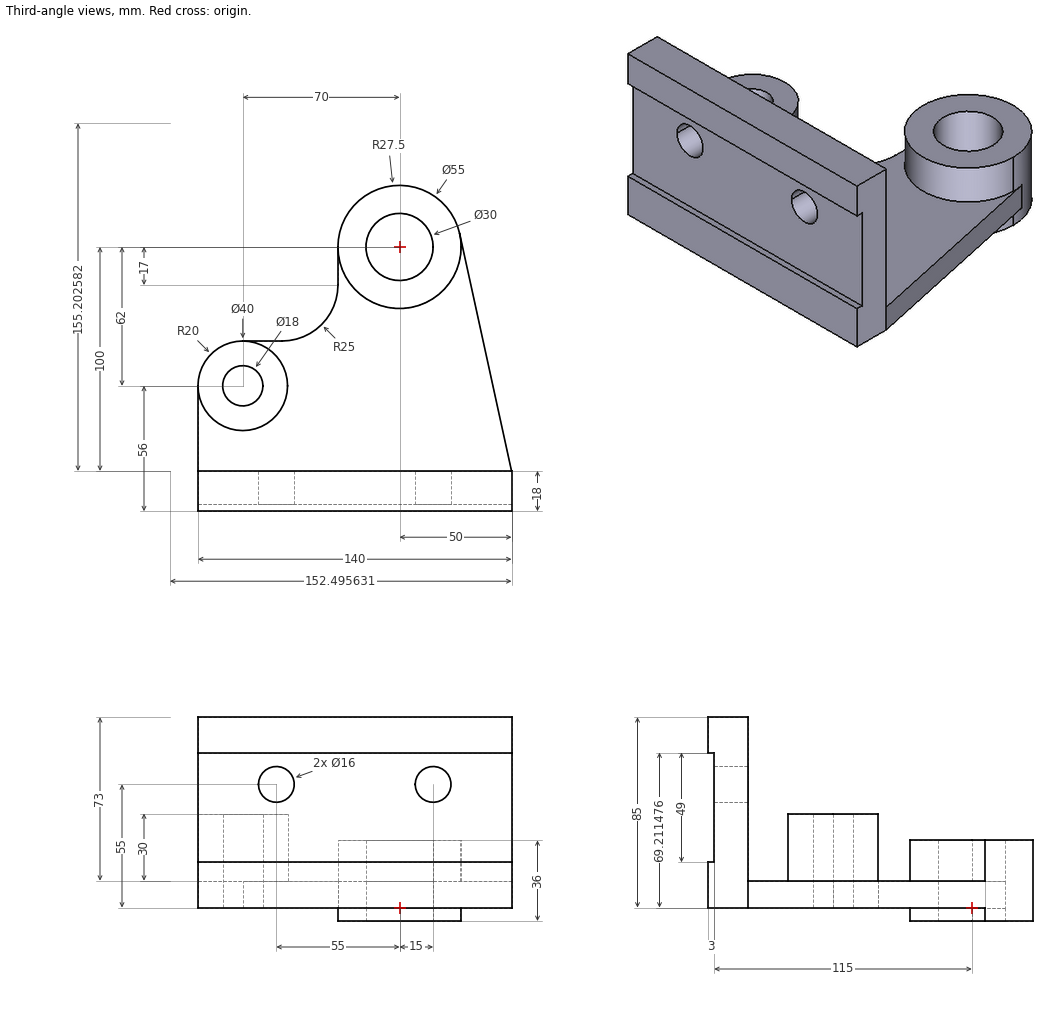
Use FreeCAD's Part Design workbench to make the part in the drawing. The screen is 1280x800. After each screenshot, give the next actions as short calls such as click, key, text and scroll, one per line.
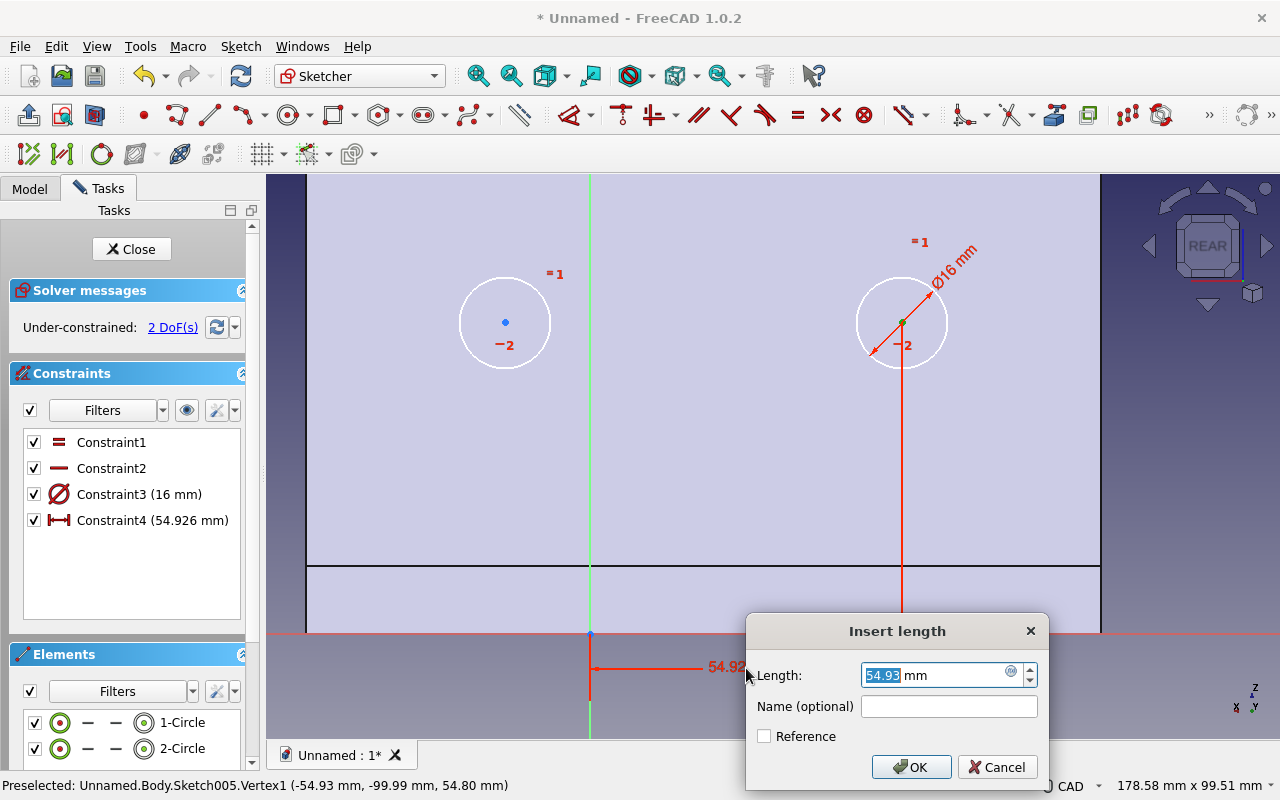
text(55)
key(Return)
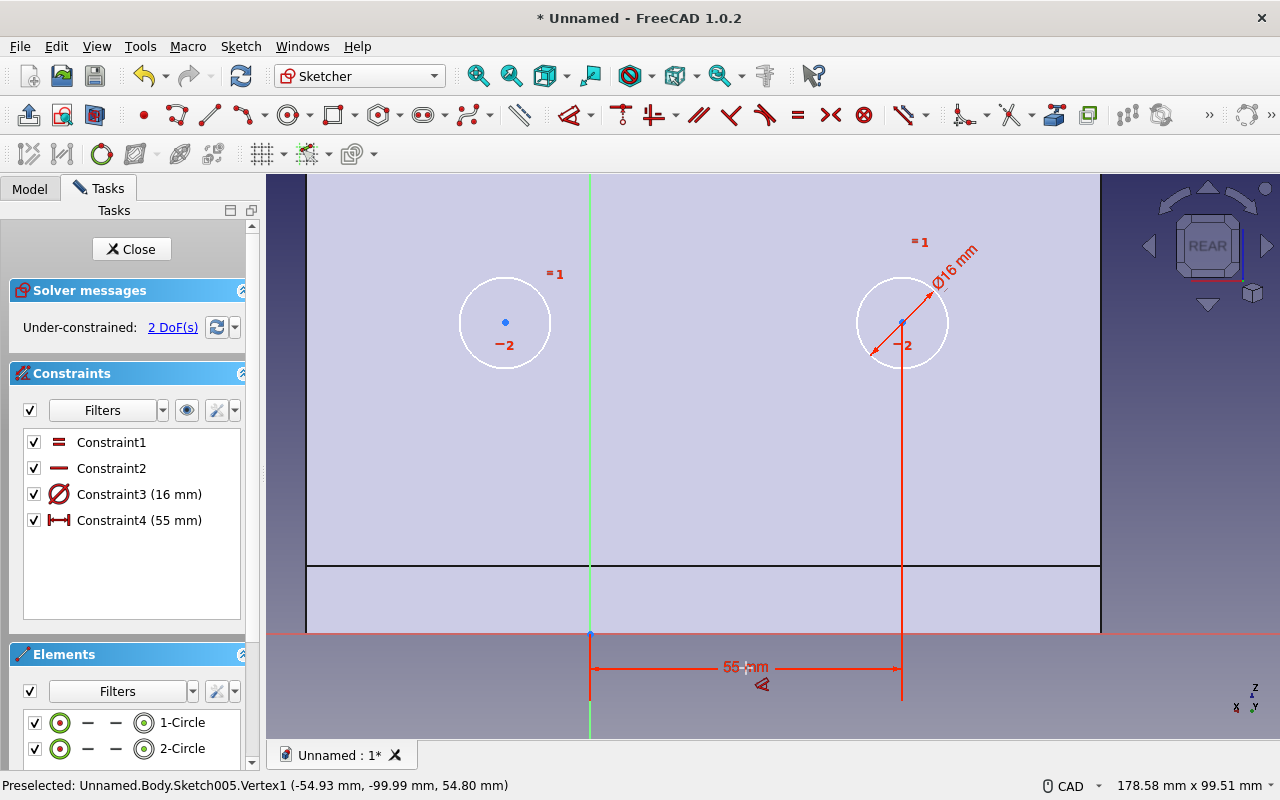
click(902, 323)
click(936, 479)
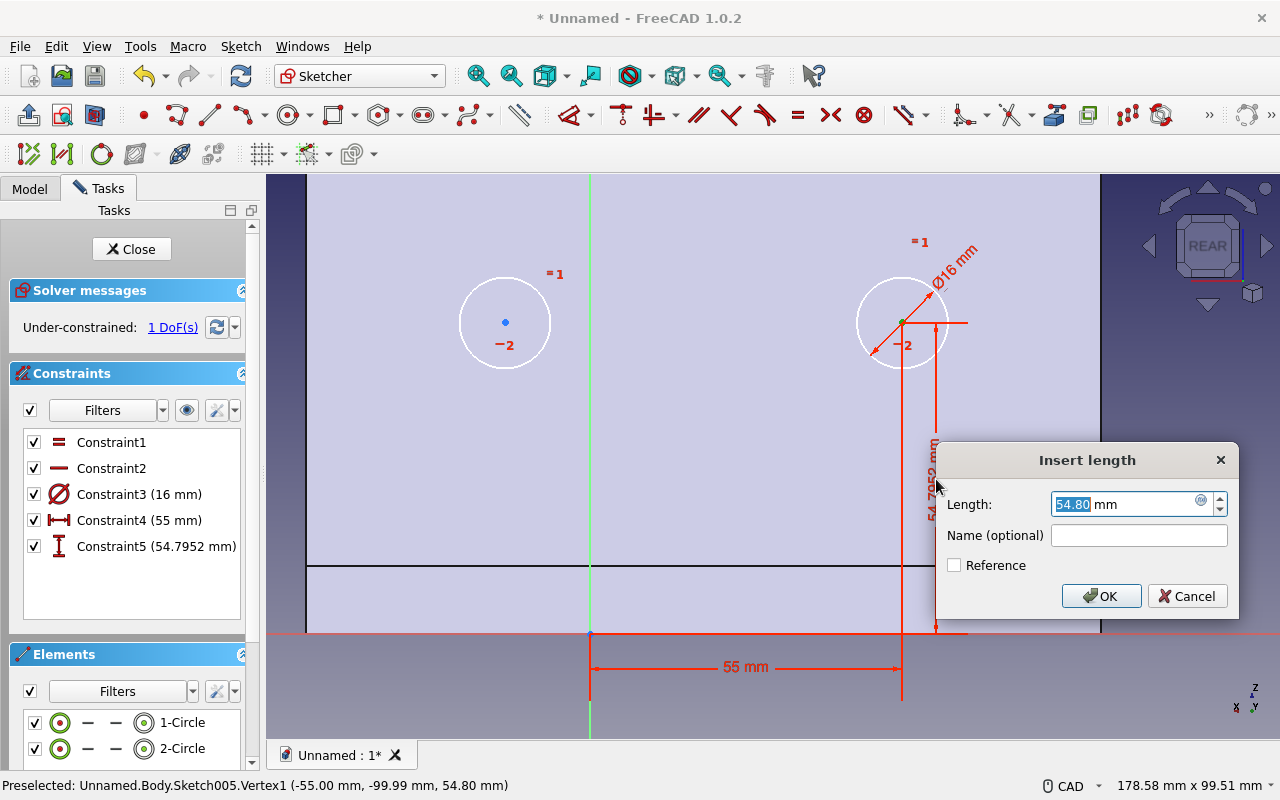
text(55)
key(Return)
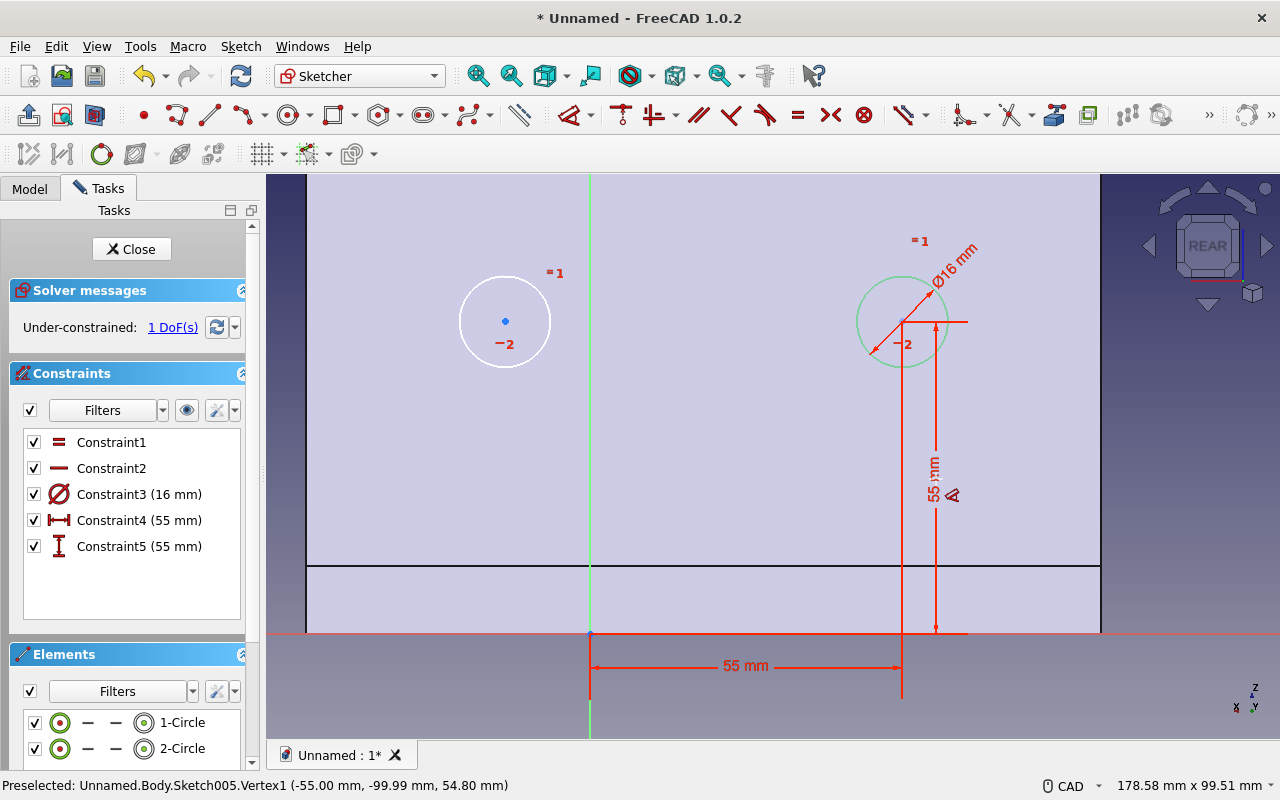
click(505, 322)
click(548, 668)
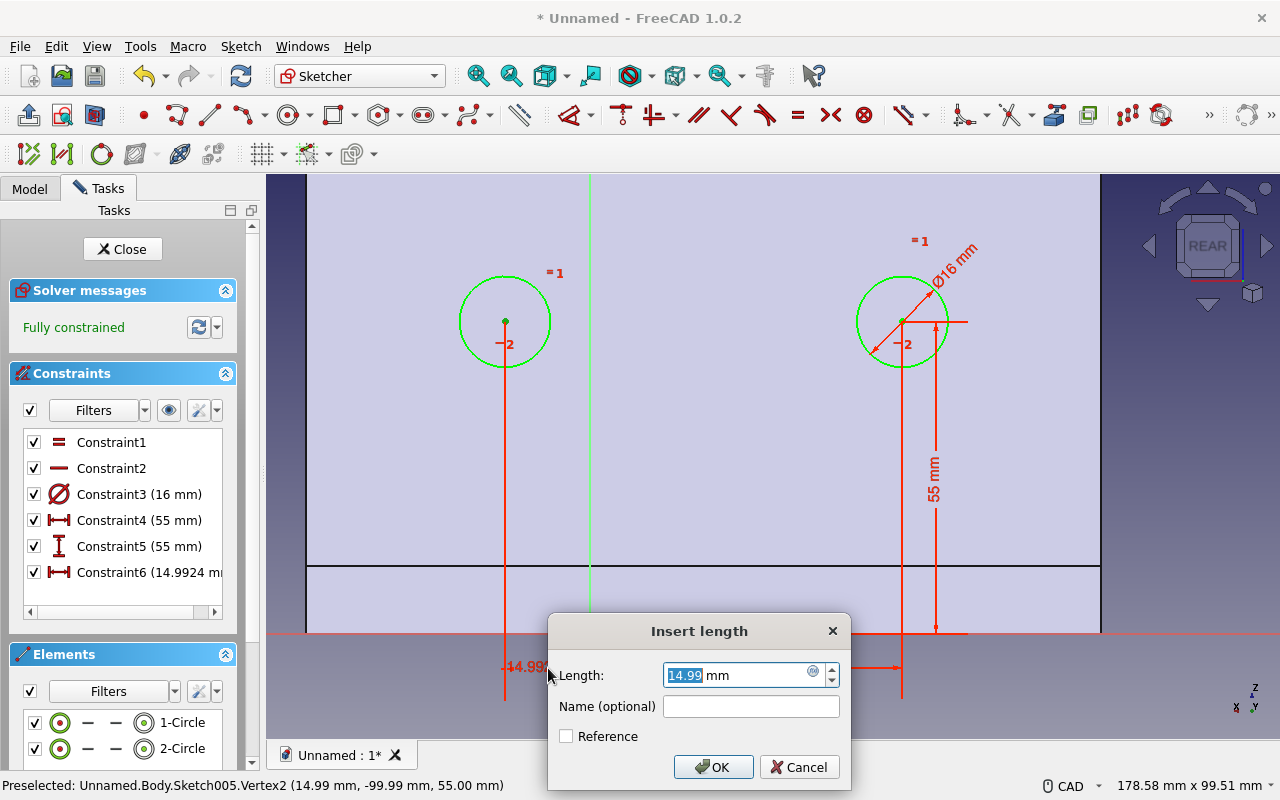
text(15)
key(Return)
key(Escape)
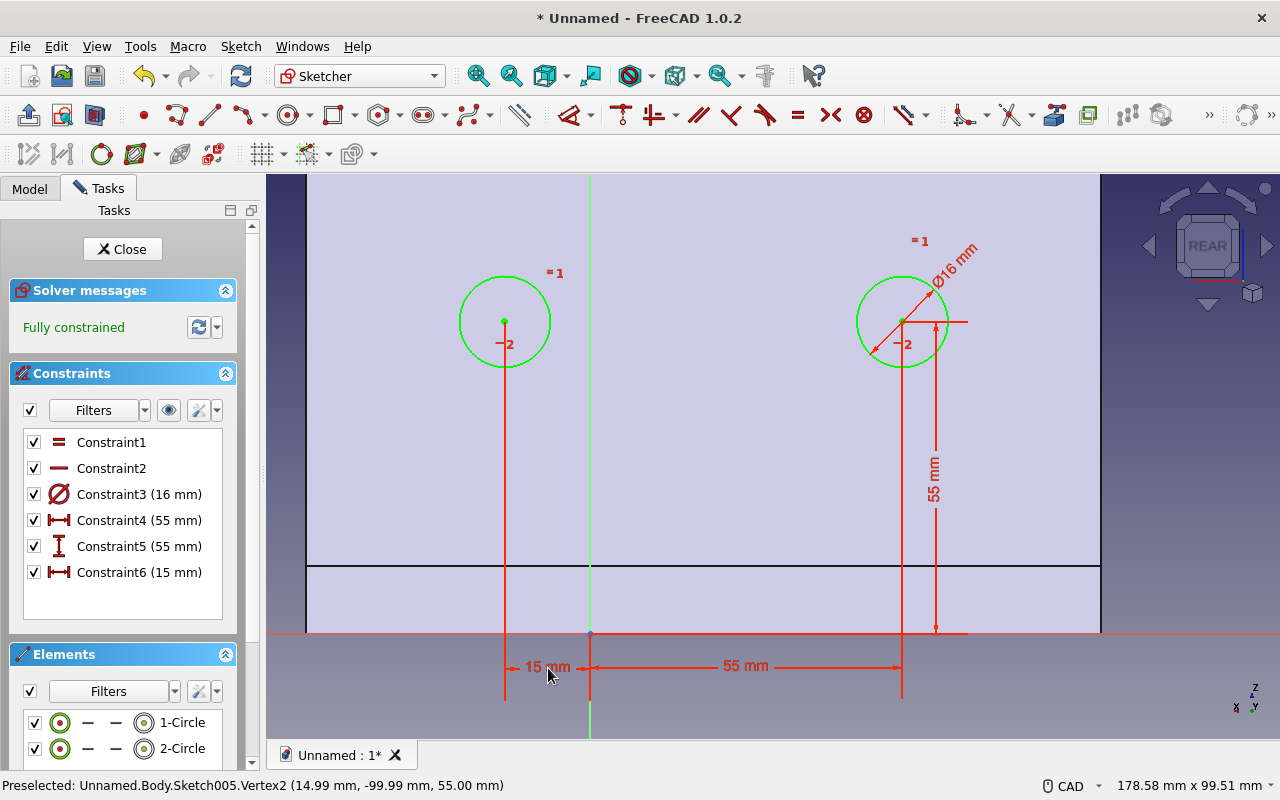
click(123, 249)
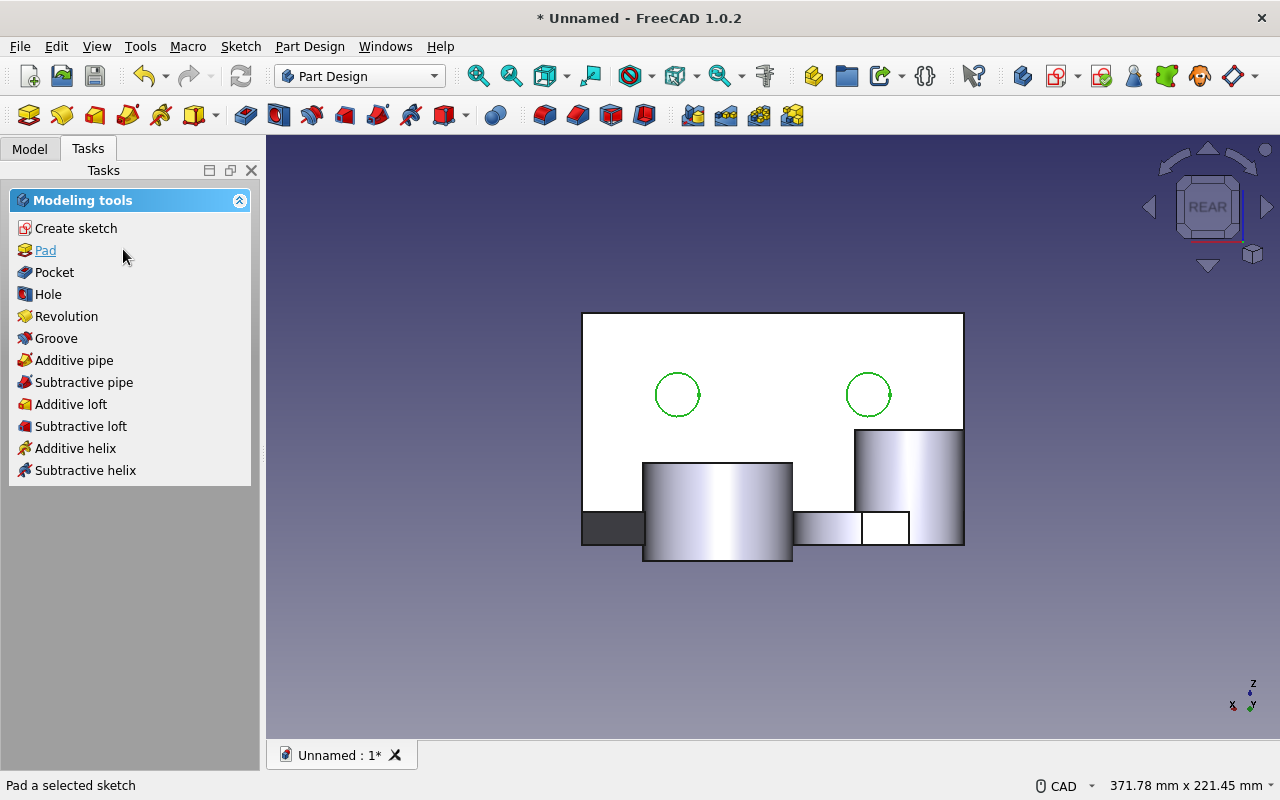
click(246, 116)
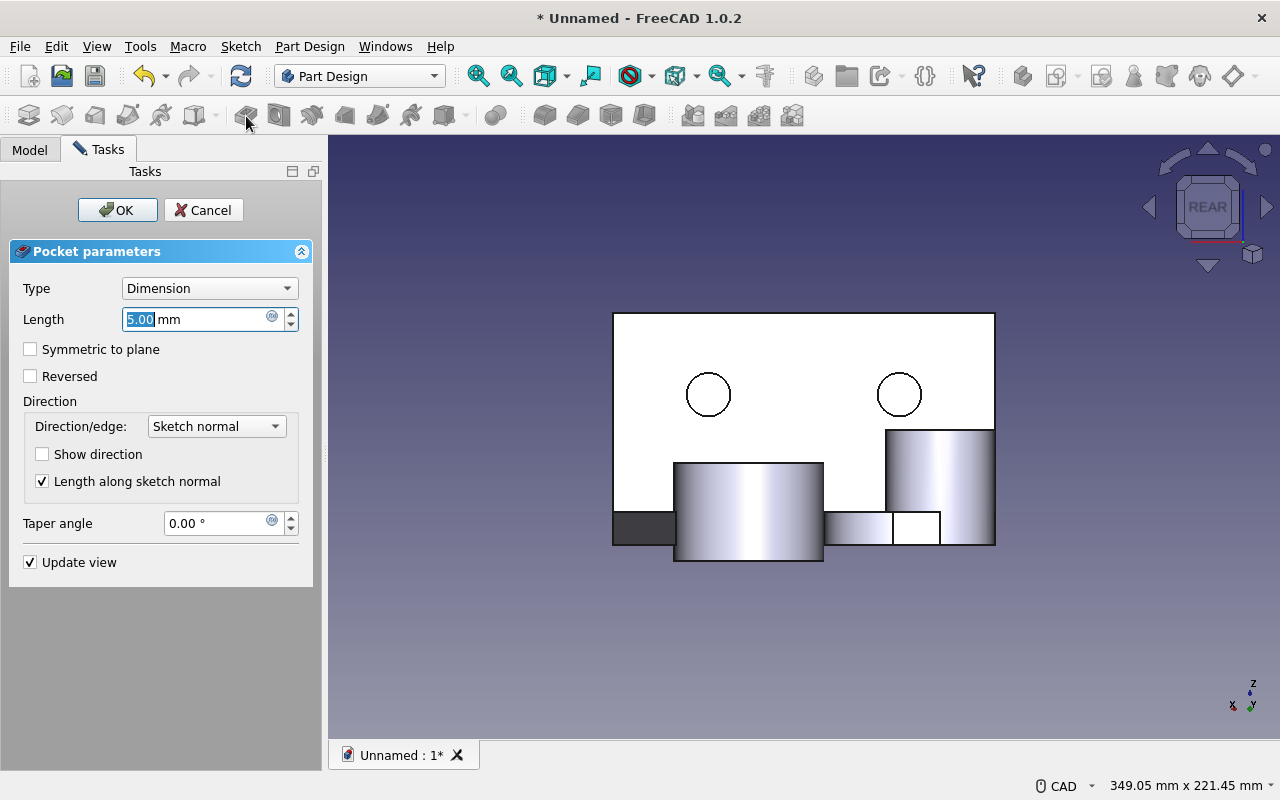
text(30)
key(Tab)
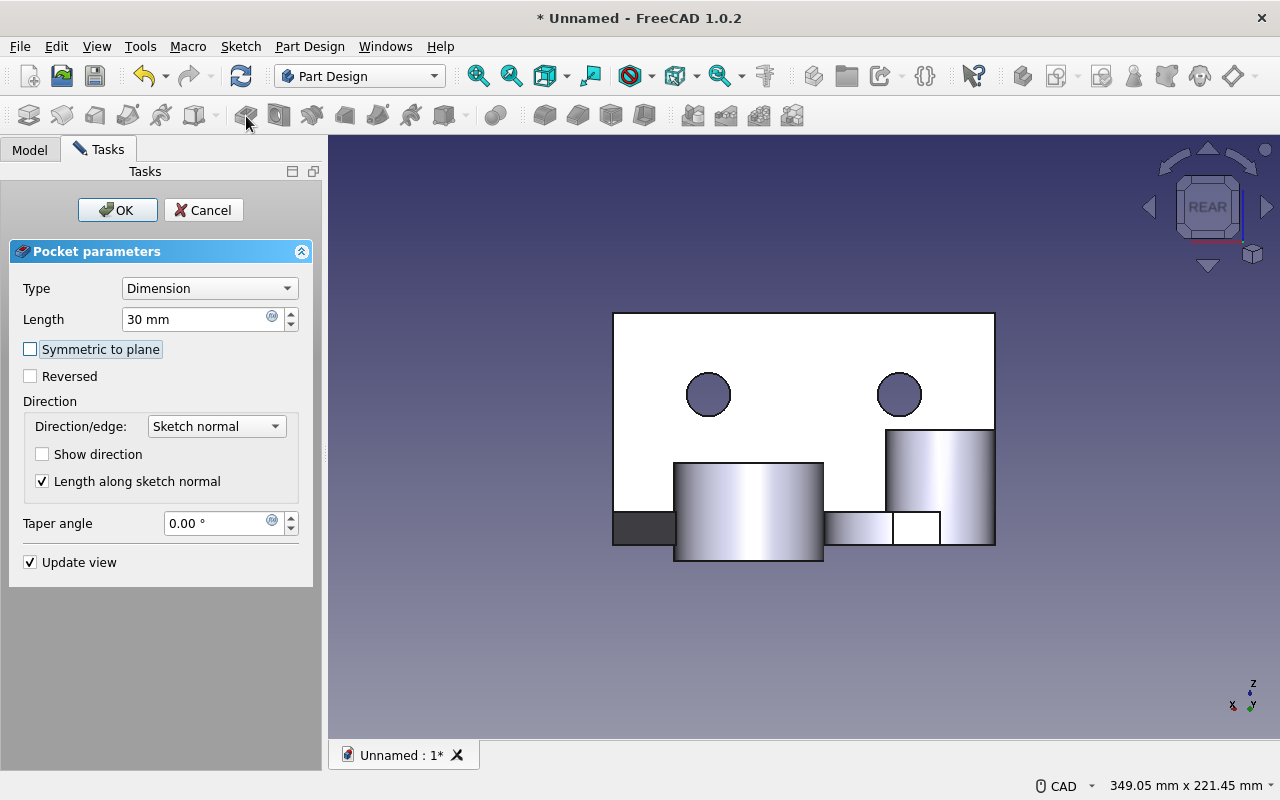
click(118, 210)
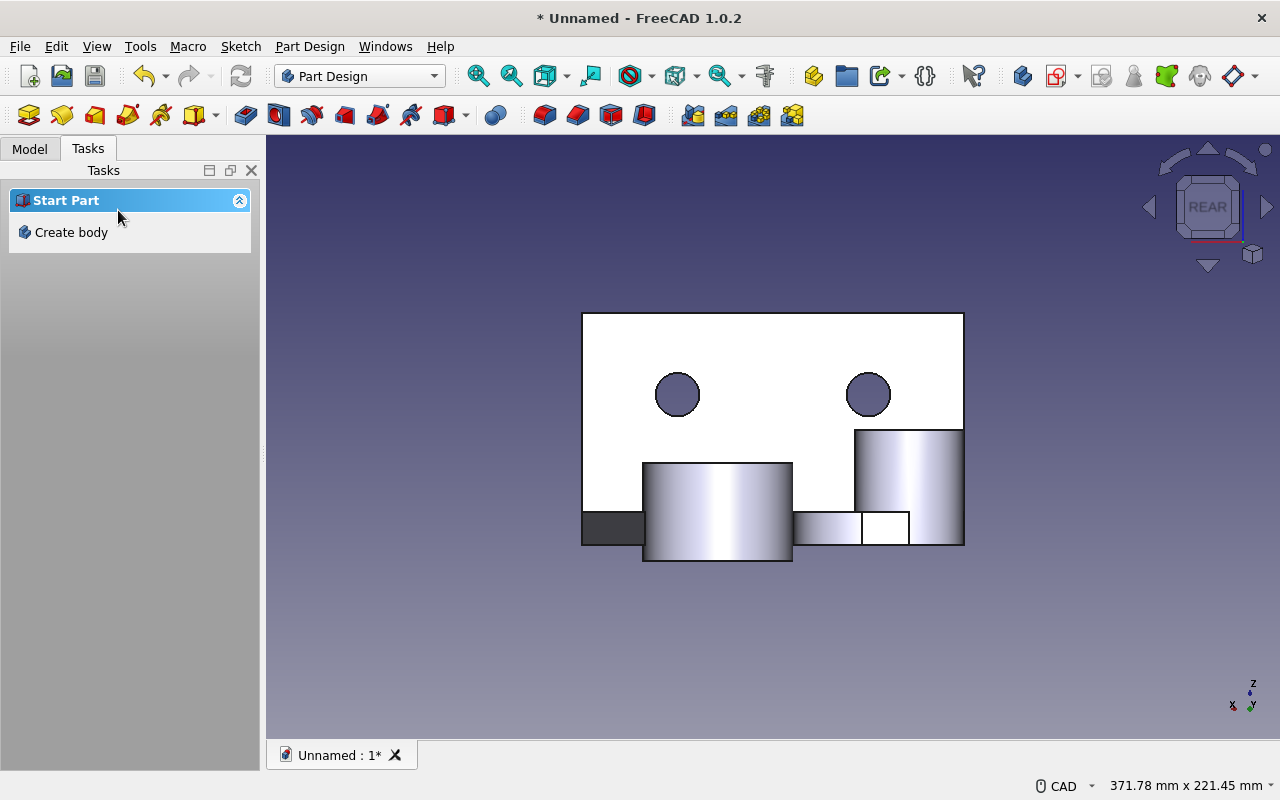
key(0)